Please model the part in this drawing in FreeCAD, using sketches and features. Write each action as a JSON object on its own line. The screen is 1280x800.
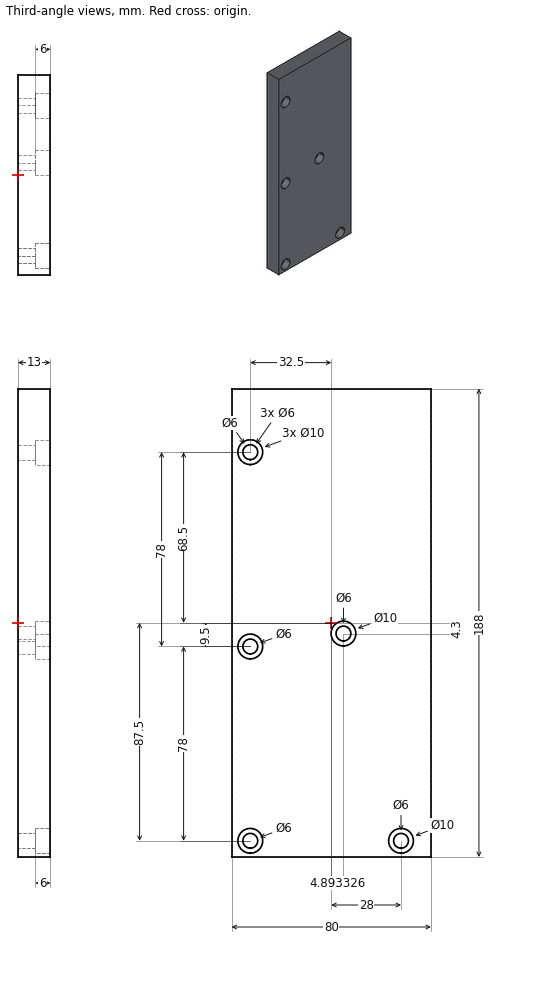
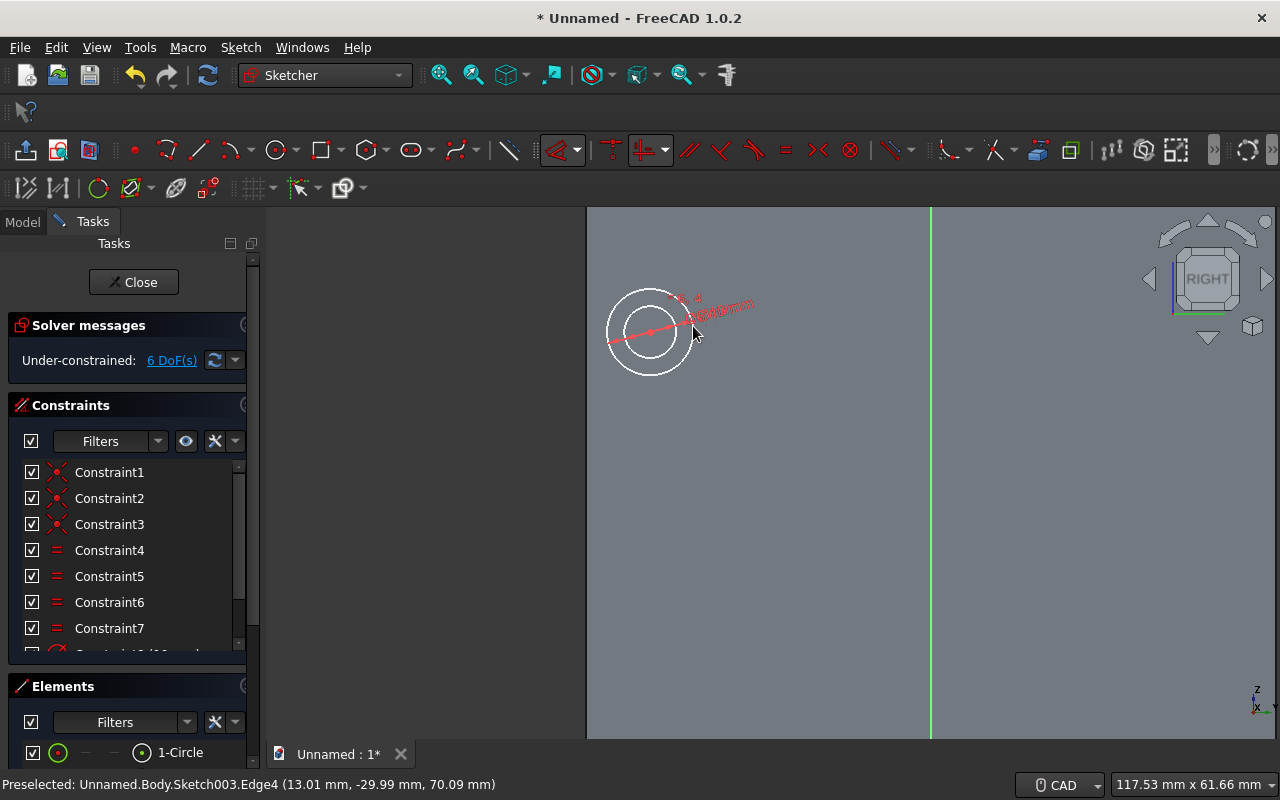
{"action": "scroll", "coordinate": [683, 300], "scroll_direction": "down", "scroll_amount": 7}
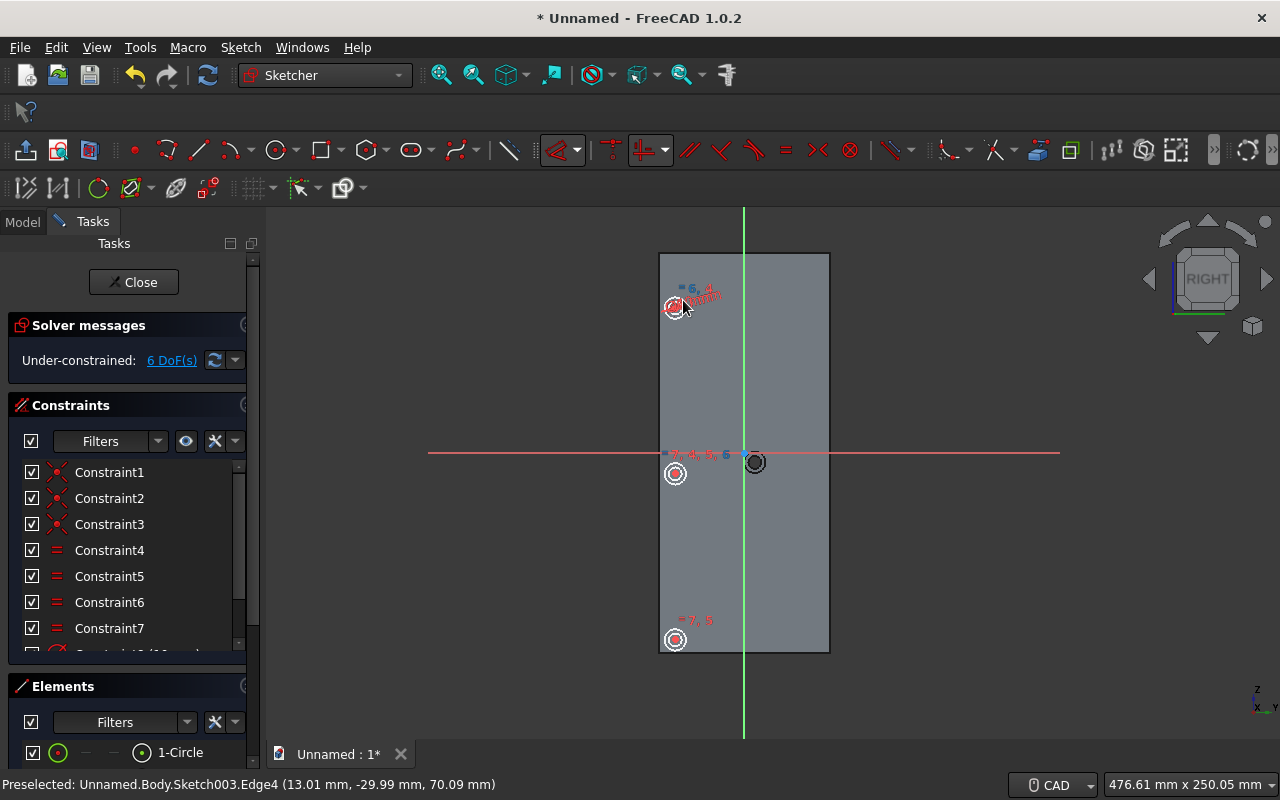
{"action": "scroll", "coordinate": [675, 474], "scroll_direction": "up", "scroll_amount": 4}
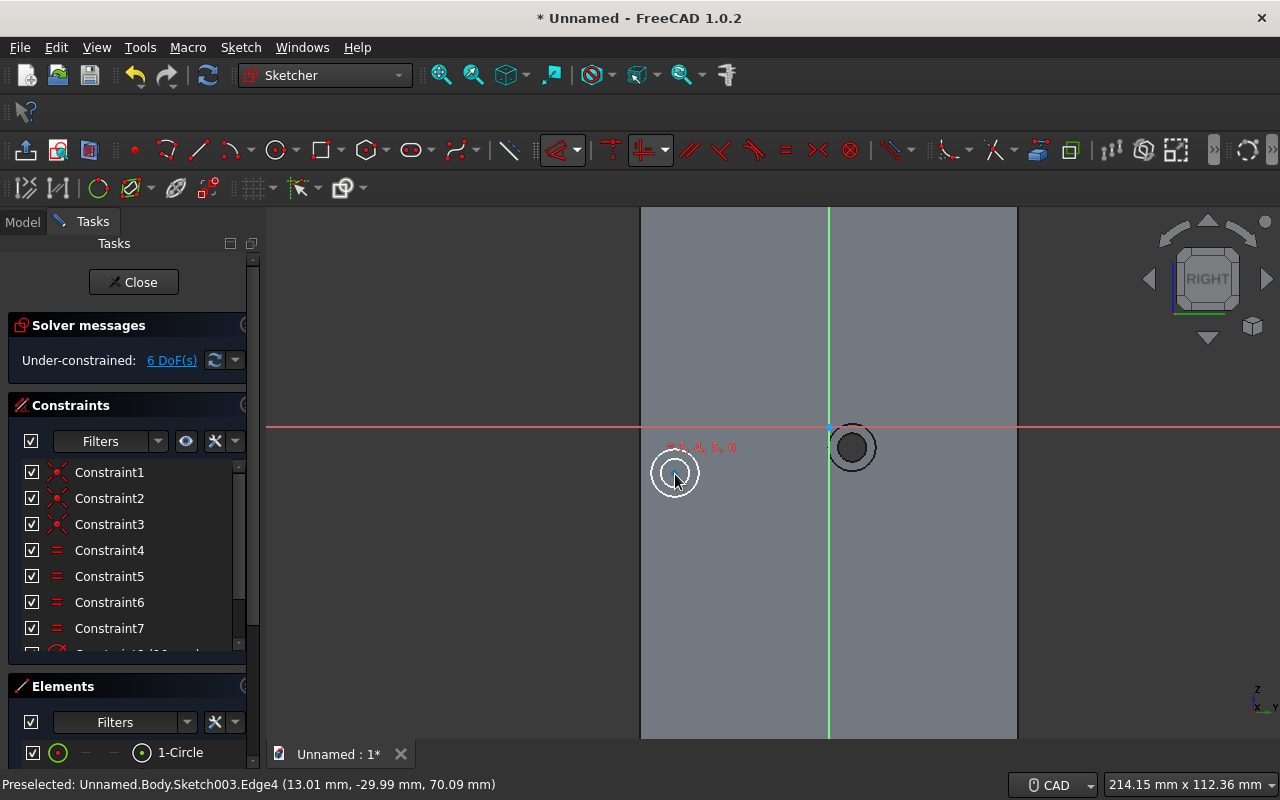
{"action": "left_click", "coordinate": [675, 473]}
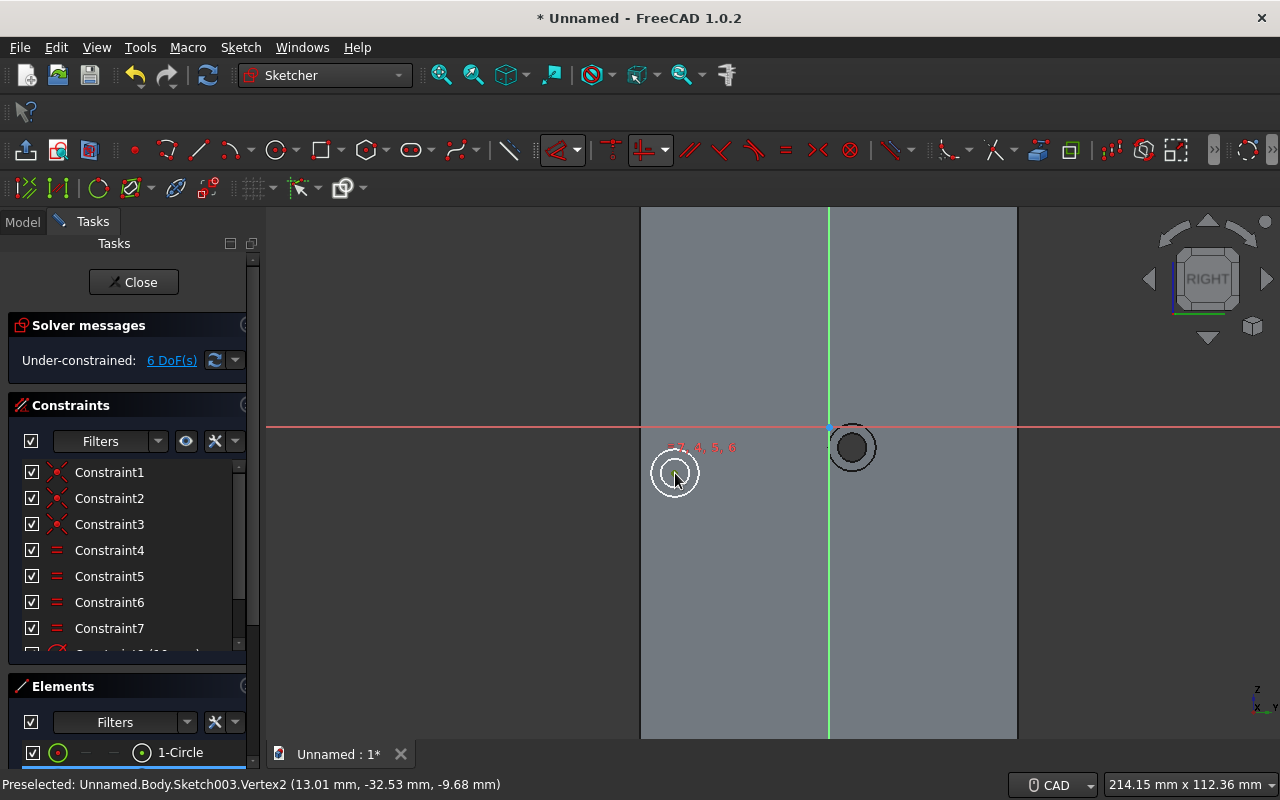
{"action": "left_click", "coordinate": [580, 150]}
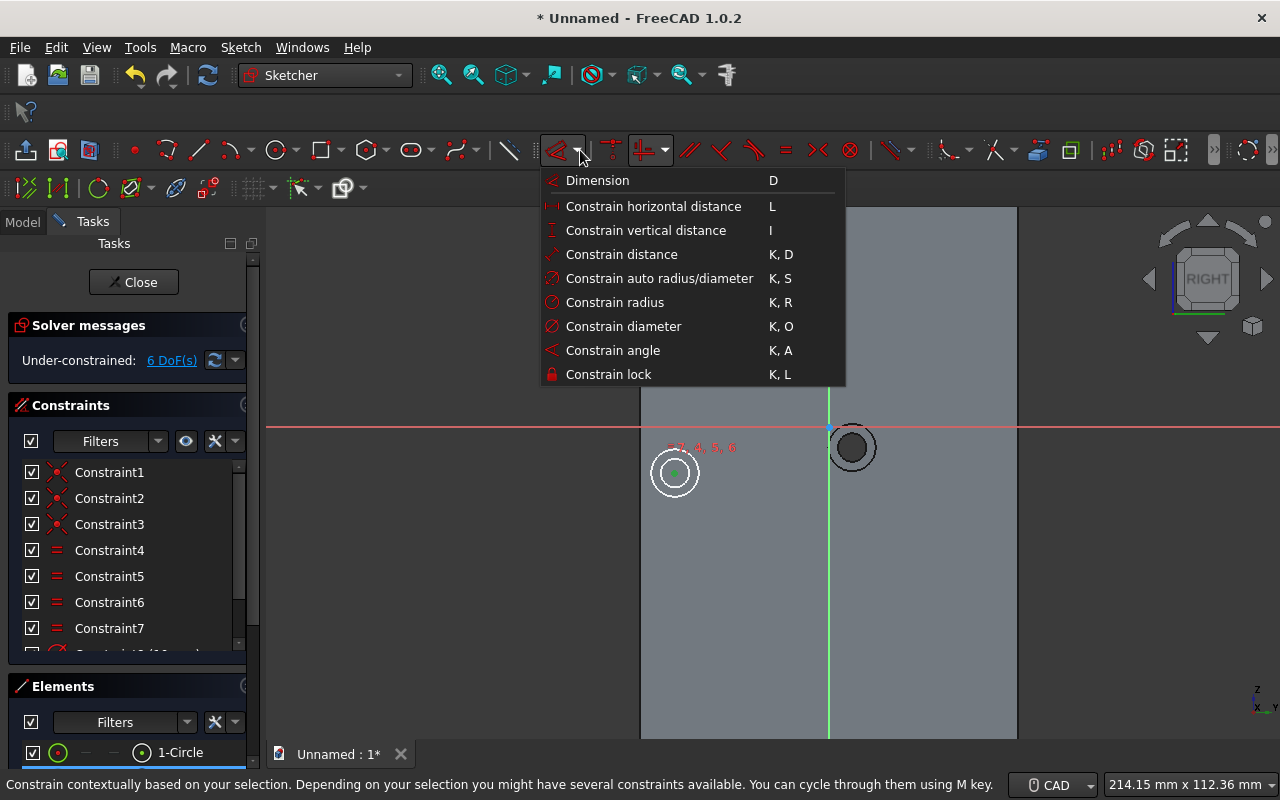
{"action": "left_click", "coordinate": [693, 230]}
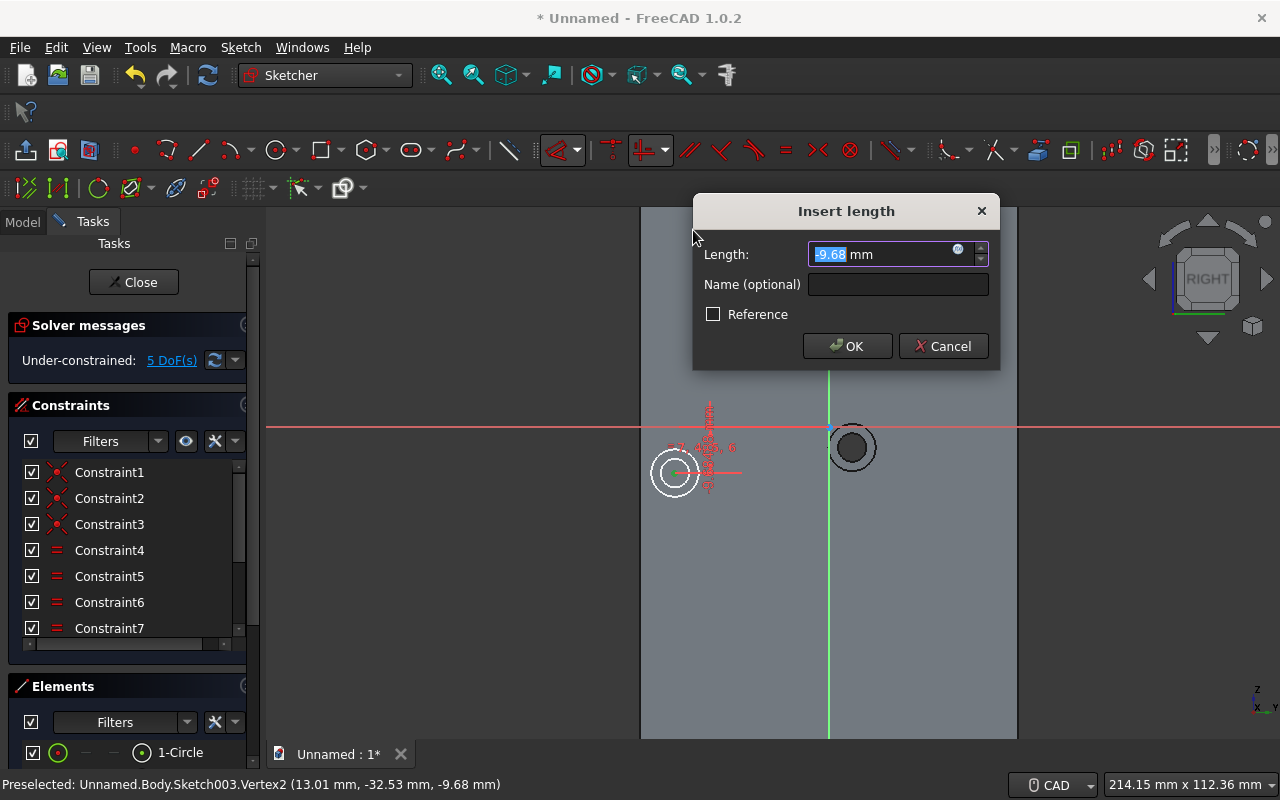
{"action": "type", "text": "-9.5"}
{"action": "key", "text": "Return"}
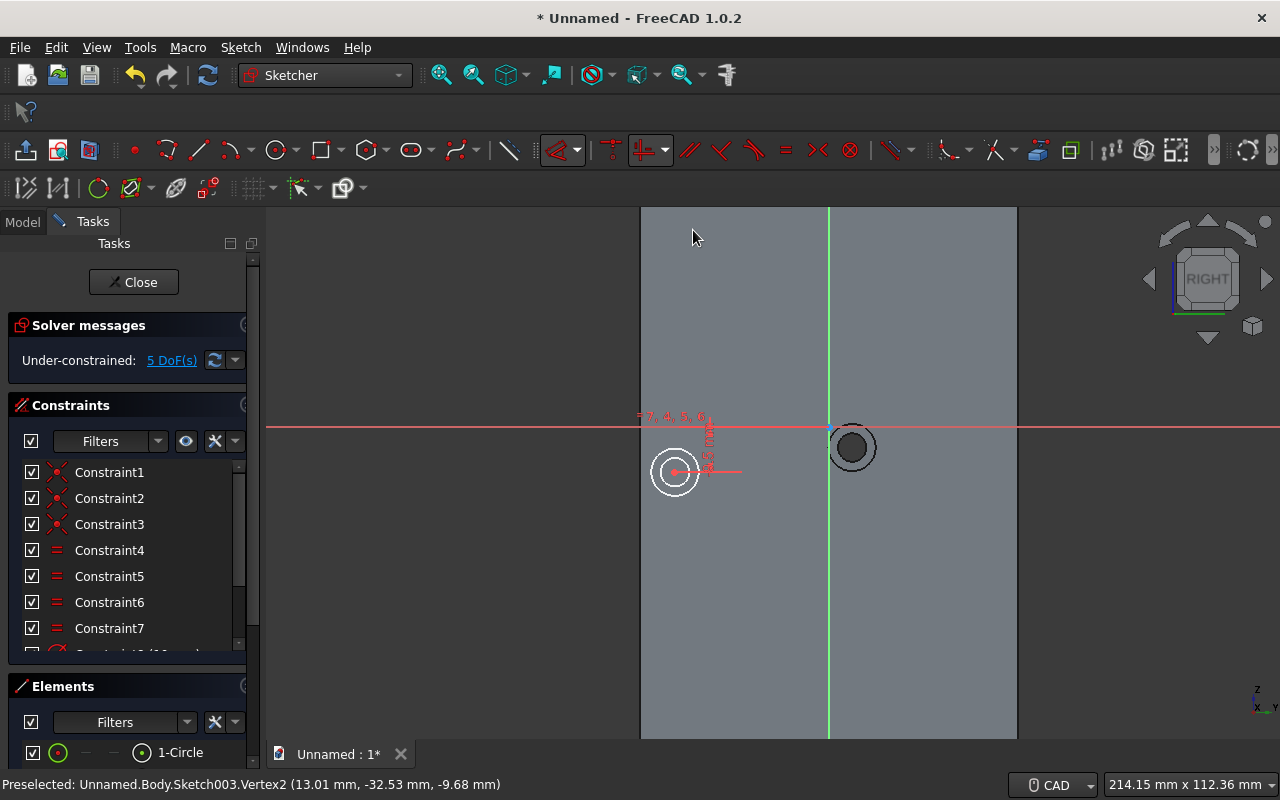
{"action": "scroll", "coordinate": [675, 474], "scroll_direction": "down", "scroll_amount": 4}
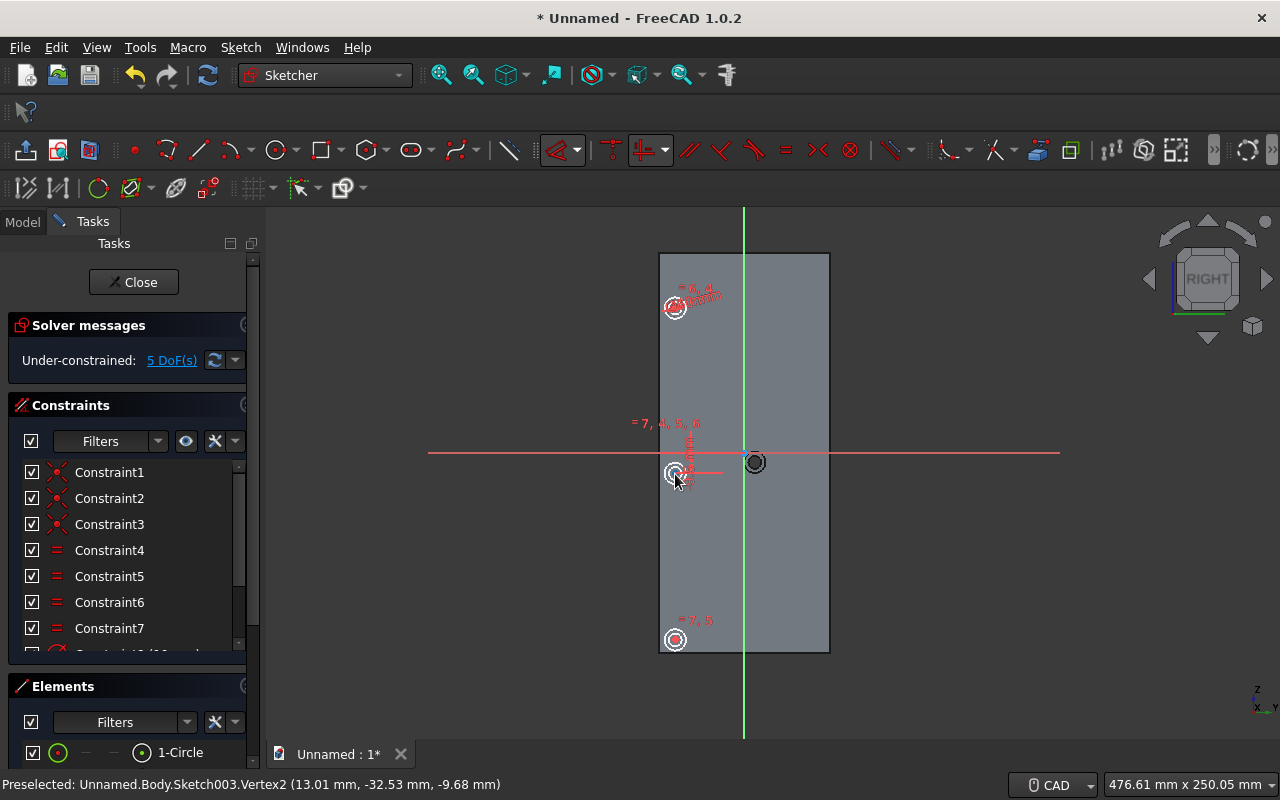
{"action": "left_click", "coordinate": [675, 308]}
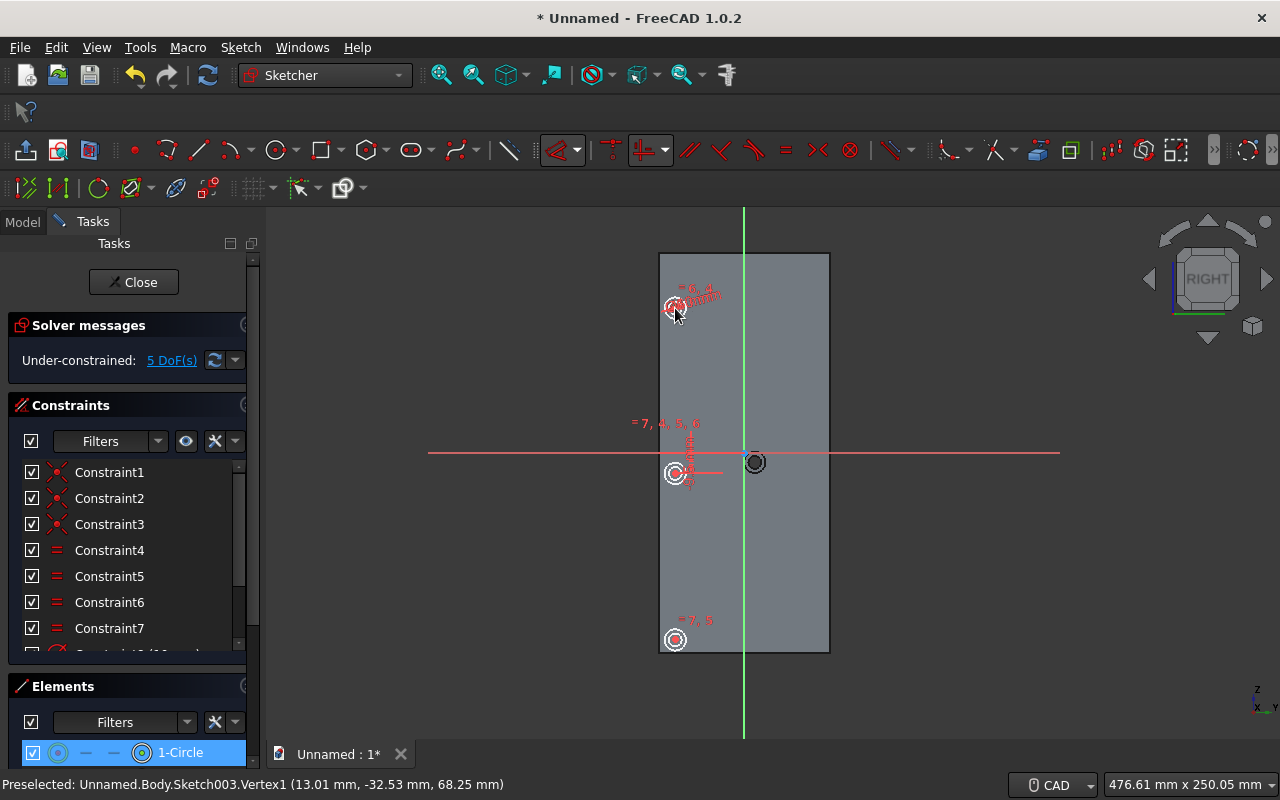
{"action": "left_click", "coordinate": [675, 473]}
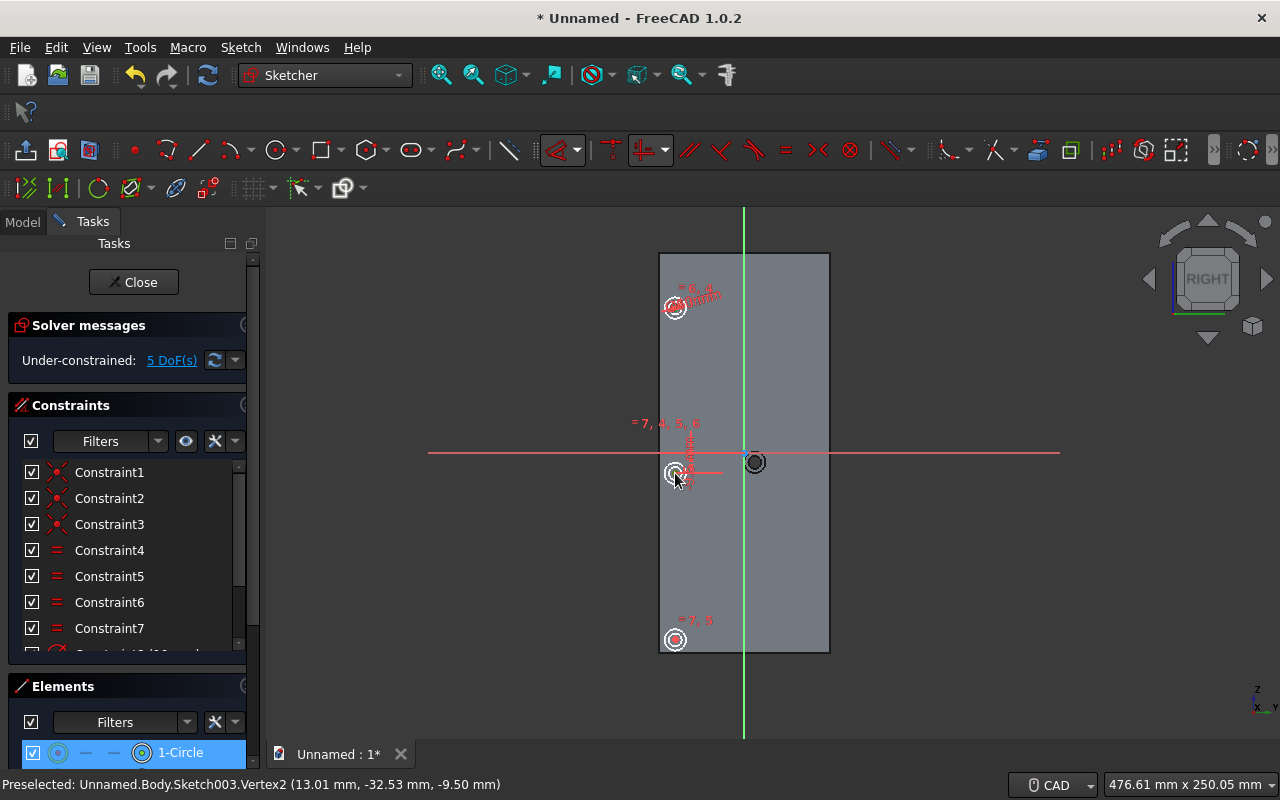
{"action": "left_click", "coordinate": [580, 150]}